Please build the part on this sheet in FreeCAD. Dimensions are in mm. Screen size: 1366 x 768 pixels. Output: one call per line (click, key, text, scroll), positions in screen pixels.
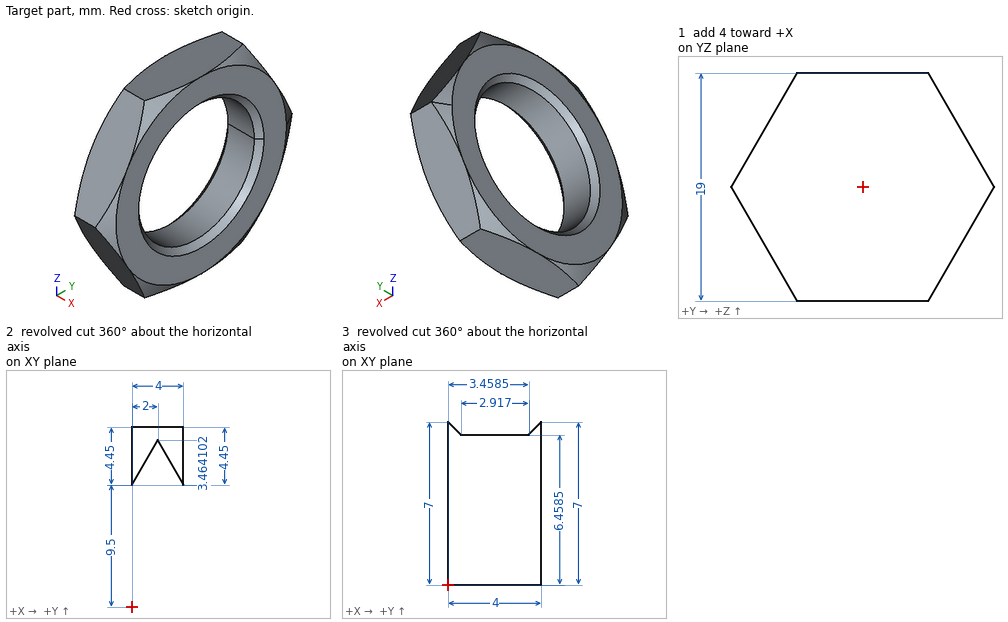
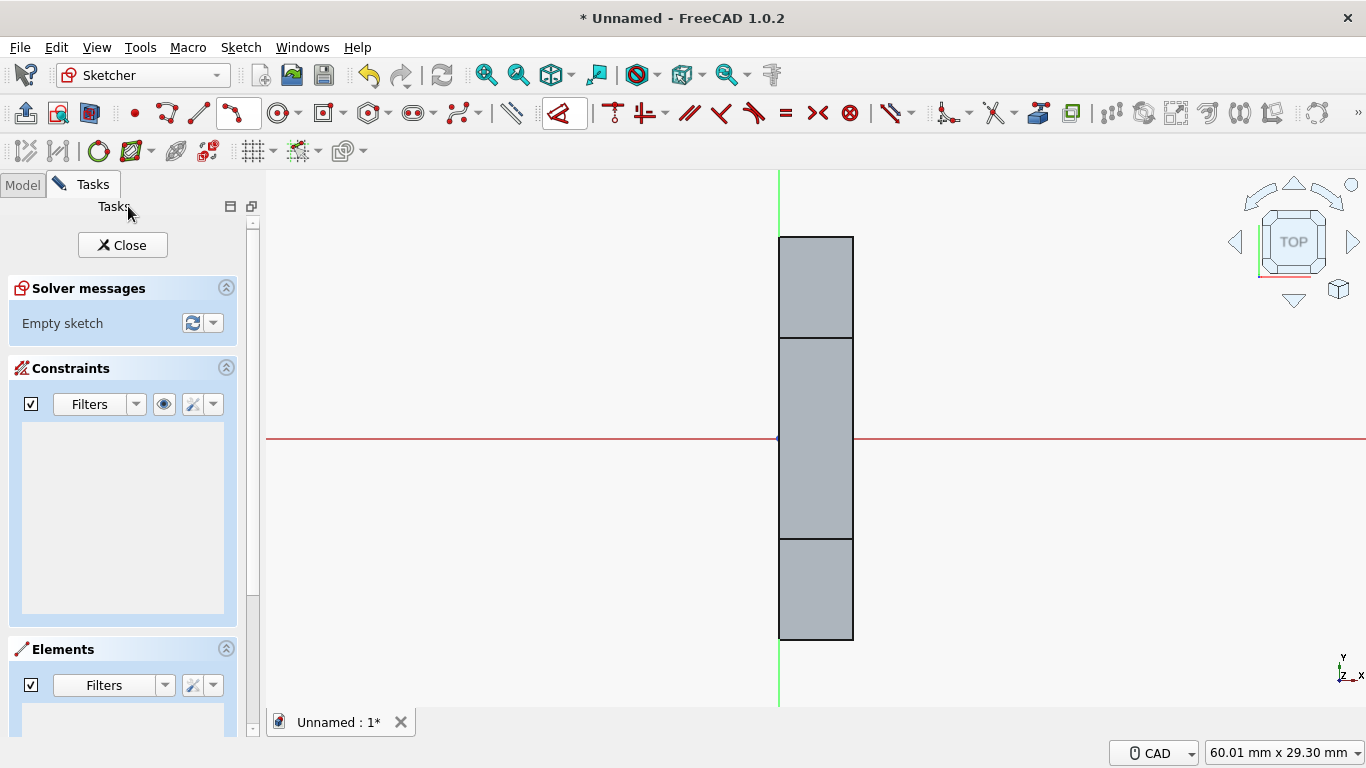
key(q)
key(s)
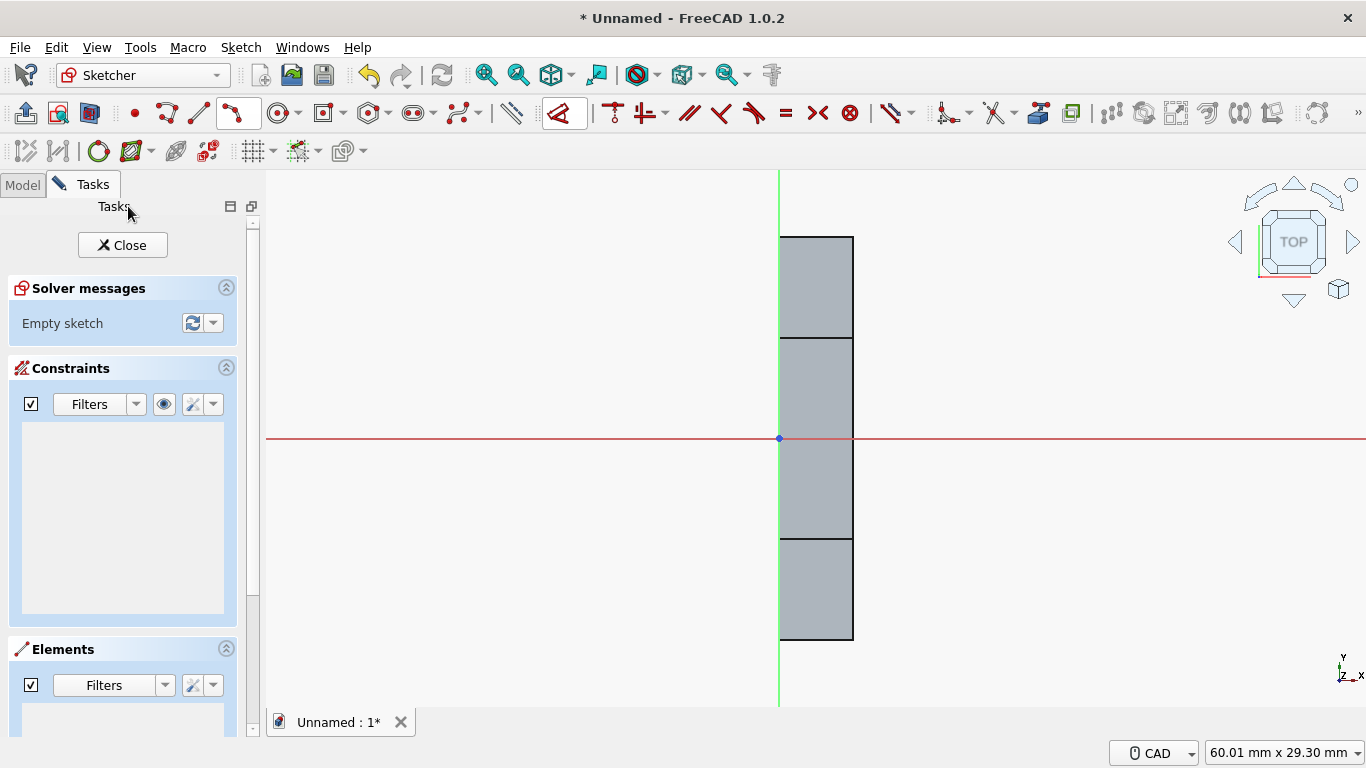
scroll(748, 438, down, 5)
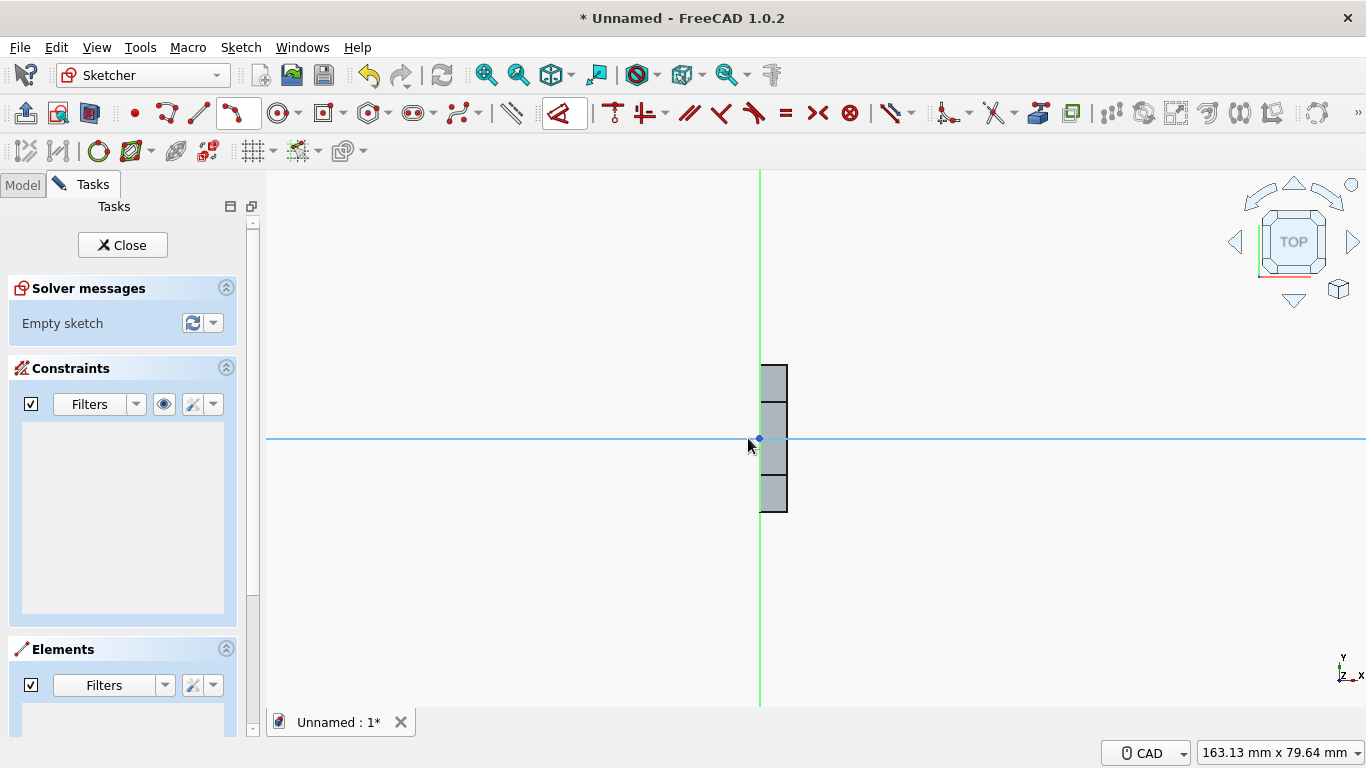
scroll(776, 352, up, 12)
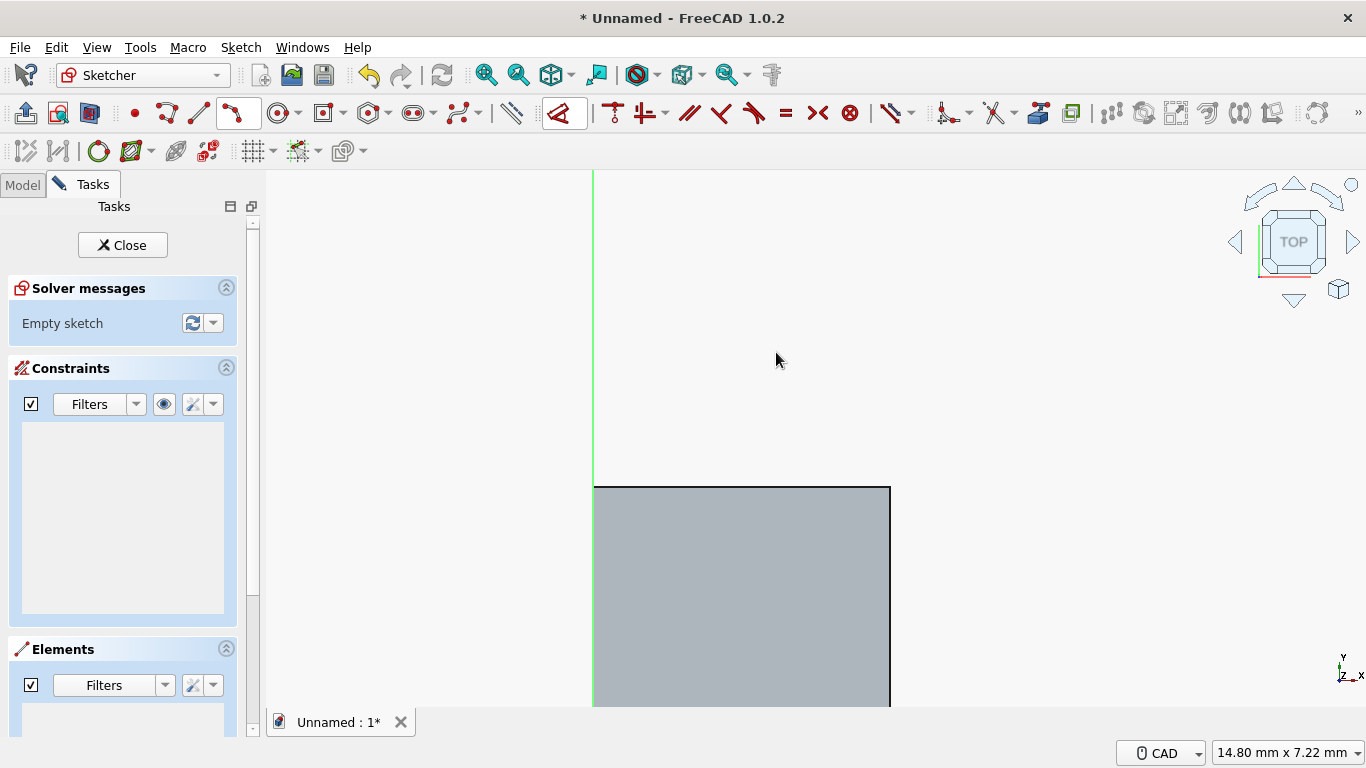
click(168, 114)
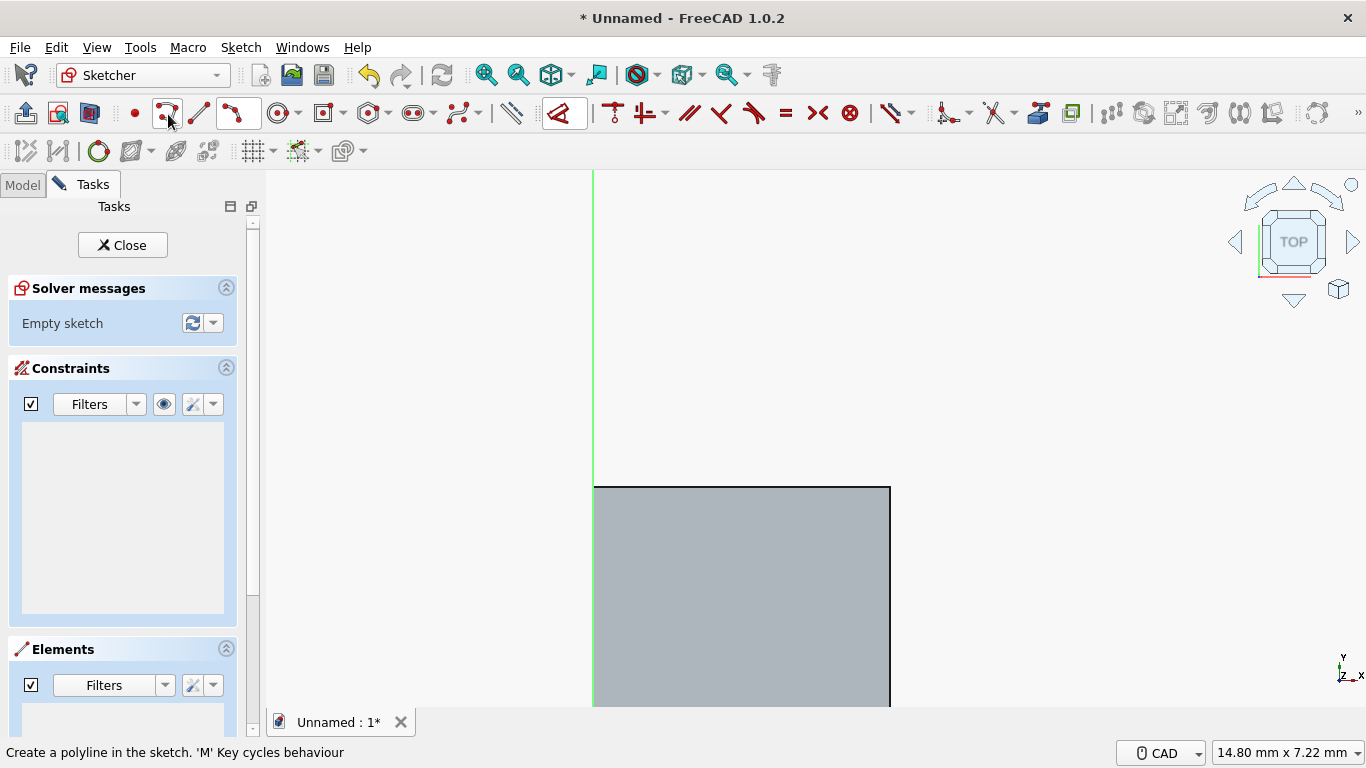
click(593, 596)
click(742, 338)
click(890, 596)
click(890, 265)
click(602, 265)
click(593, 597)
key(Escape)
key(Escape)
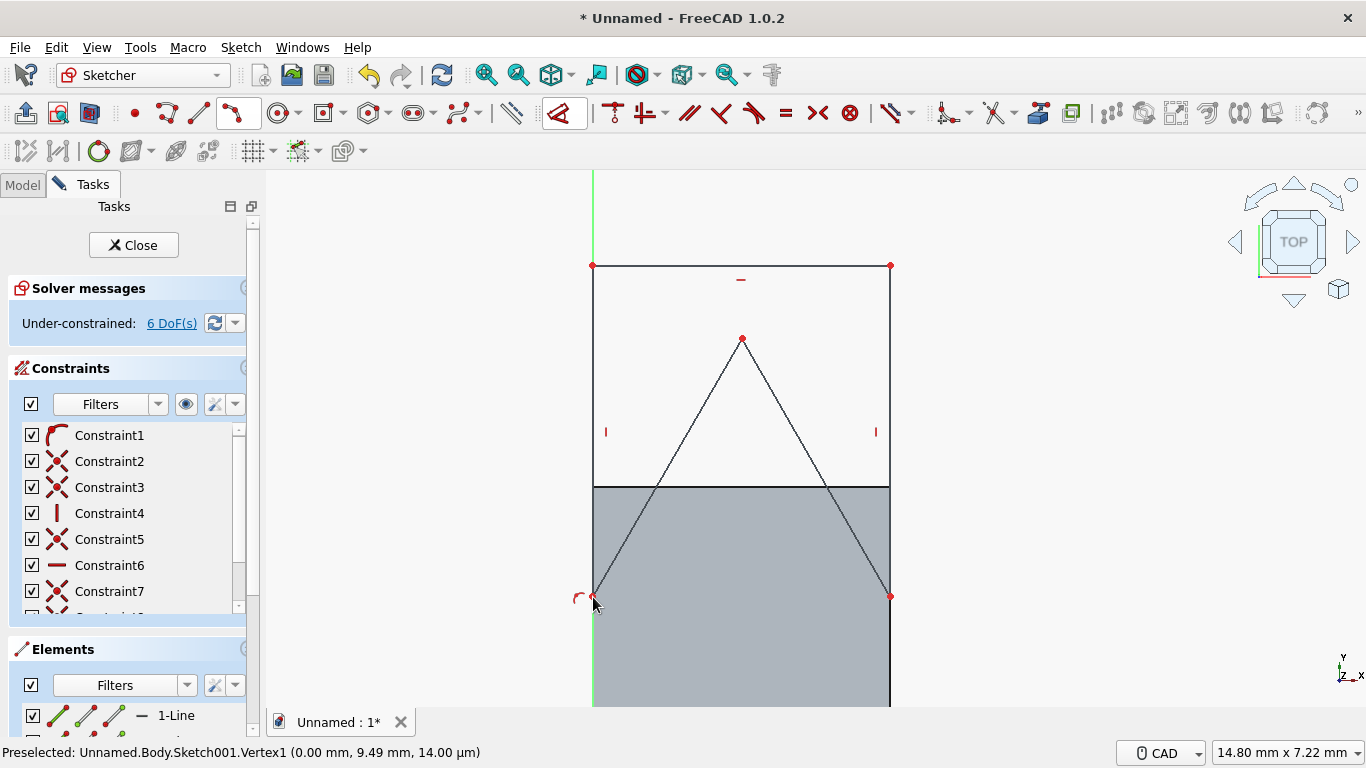
click(801, 266)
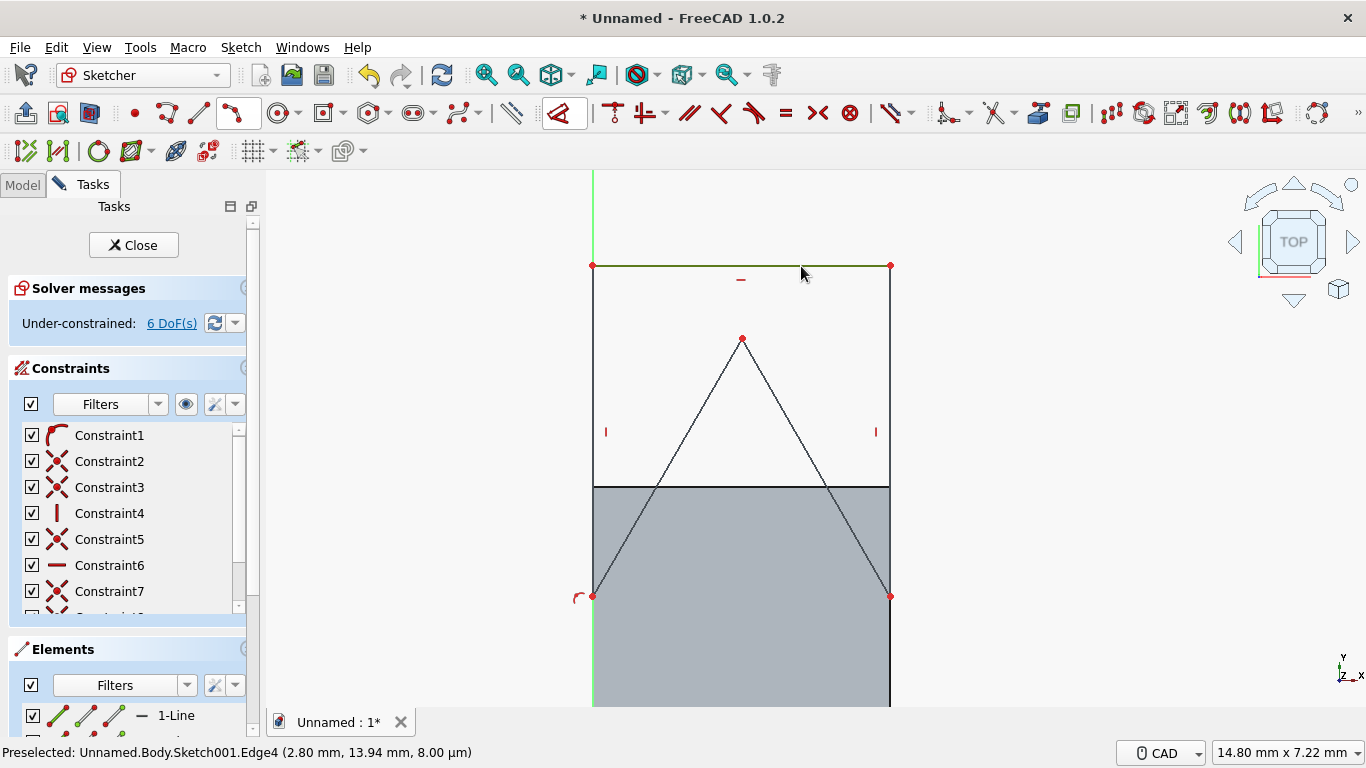
key(l)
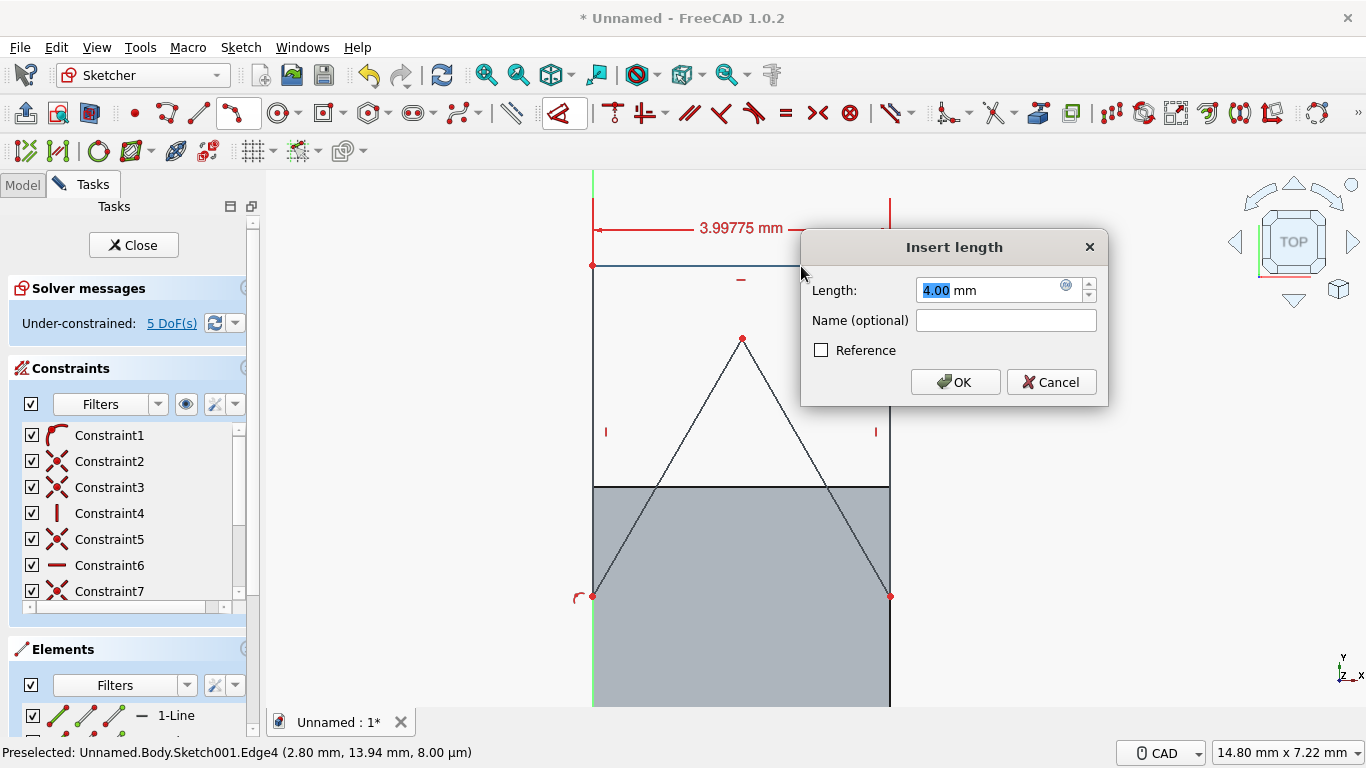
text(4)
key(Return)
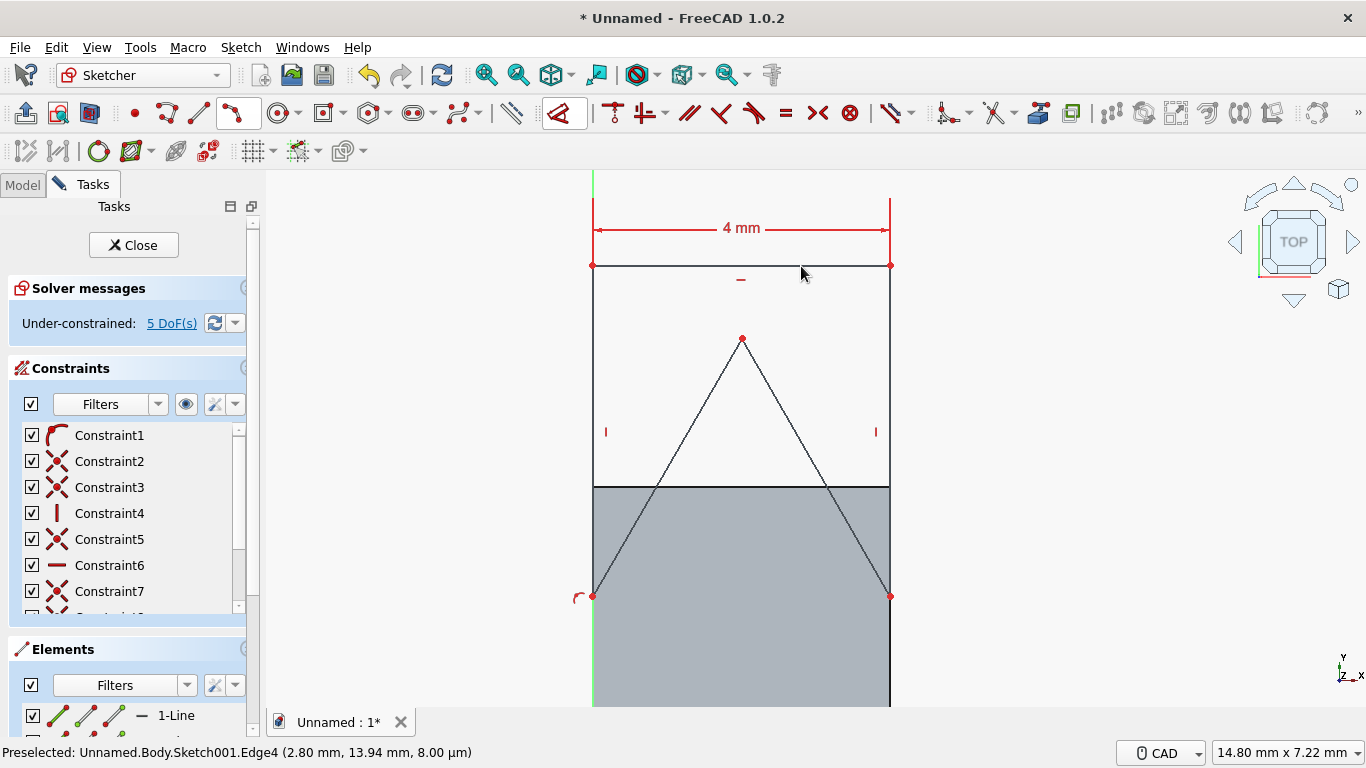
click(742, 339)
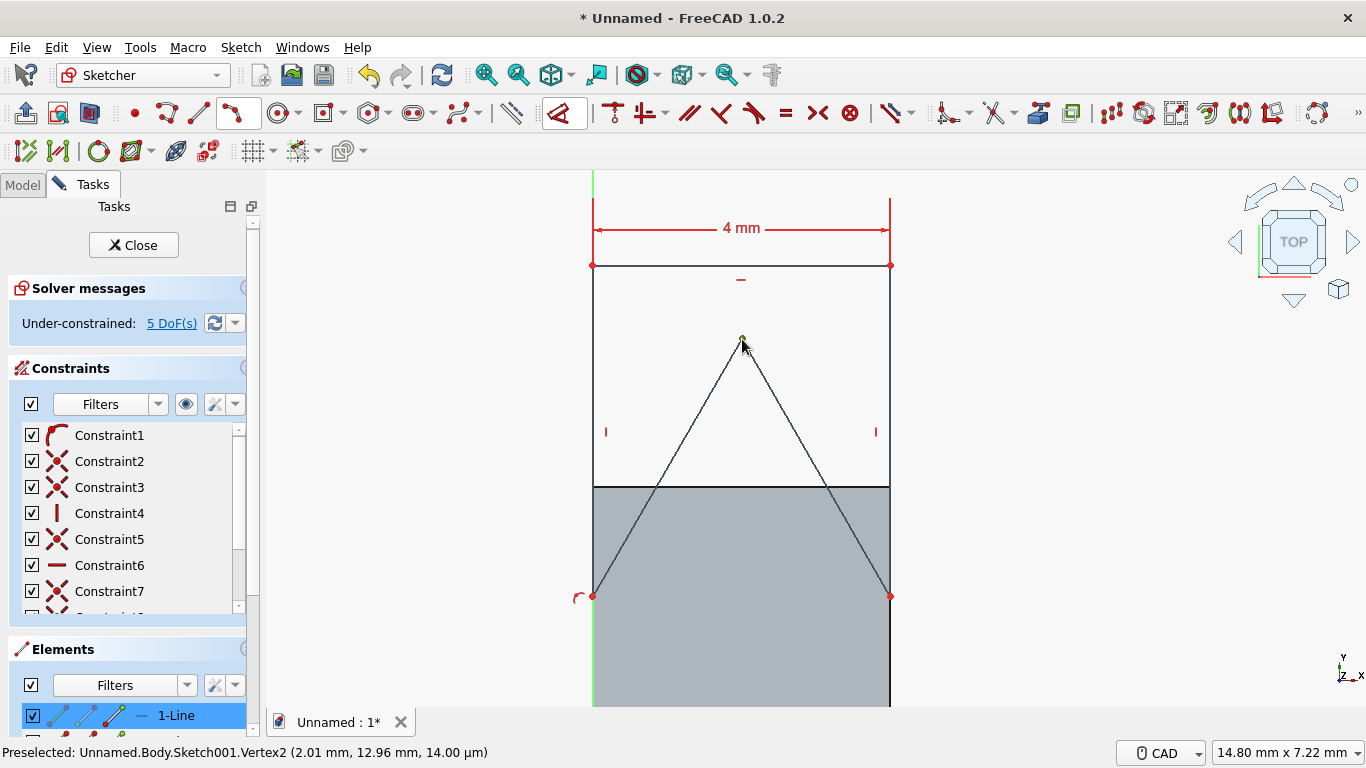
key(l)